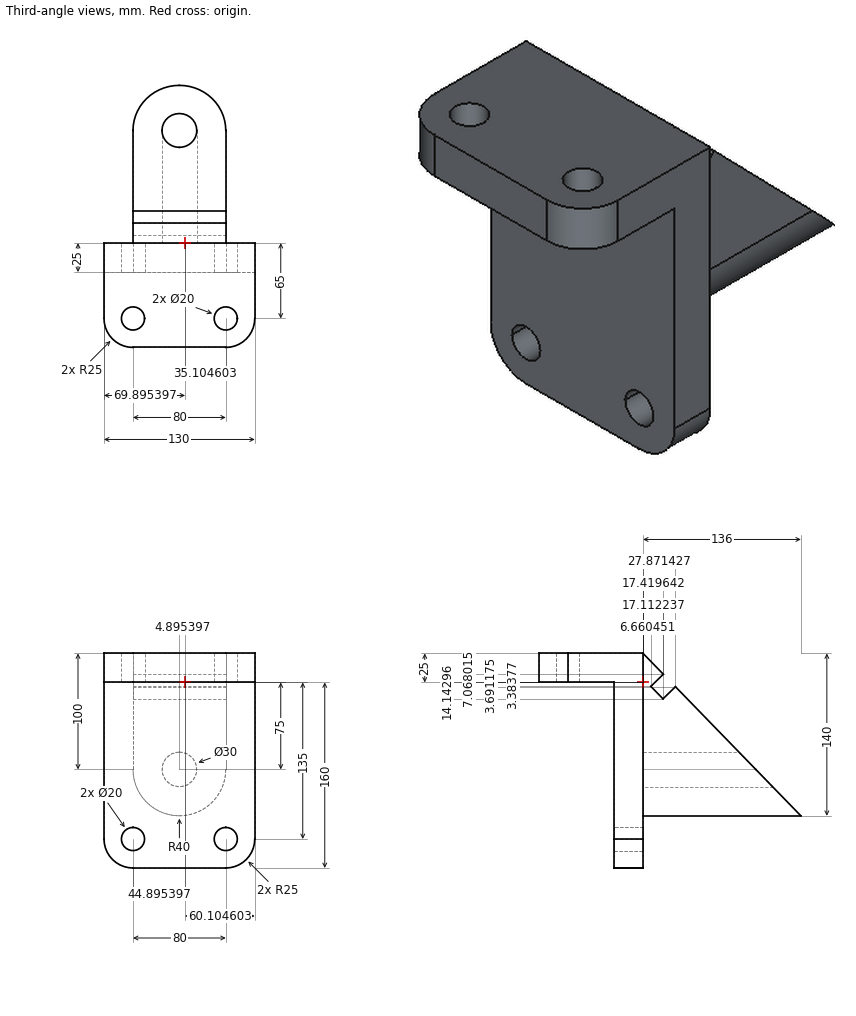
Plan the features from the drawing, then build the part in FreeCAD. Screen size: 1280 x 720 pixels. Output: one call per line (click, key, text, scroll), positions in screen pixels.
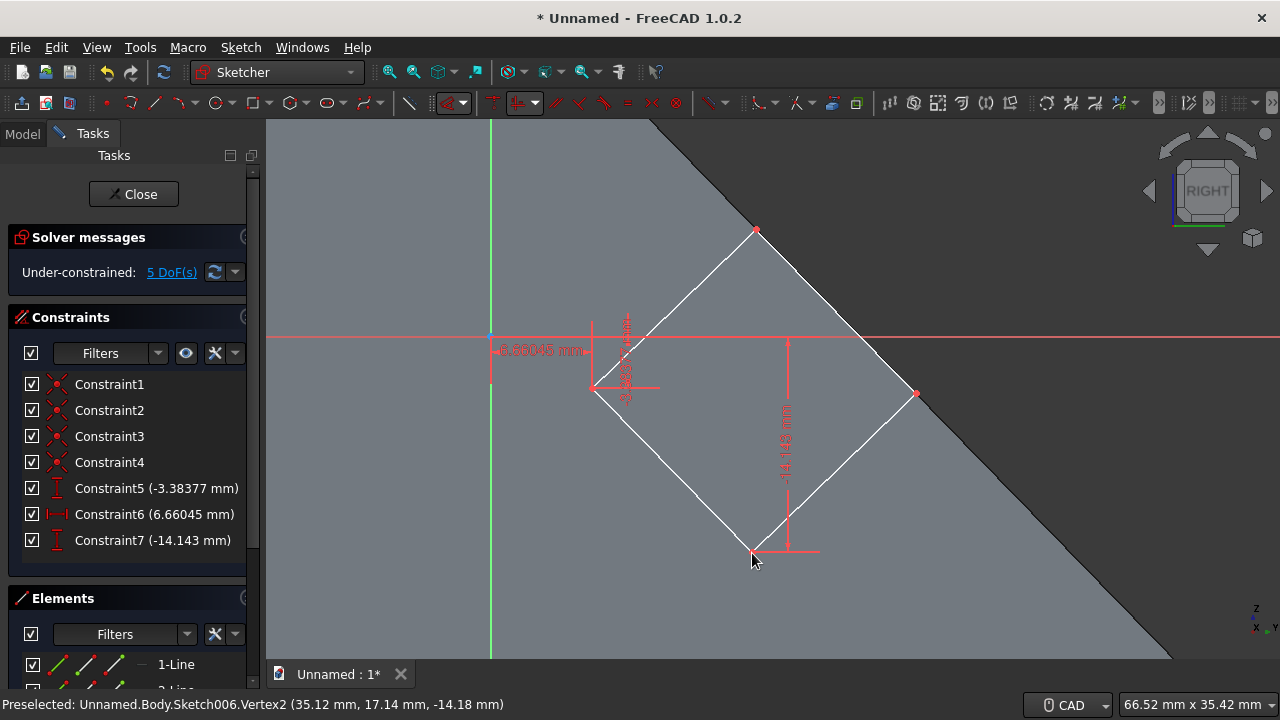
click(916, 394)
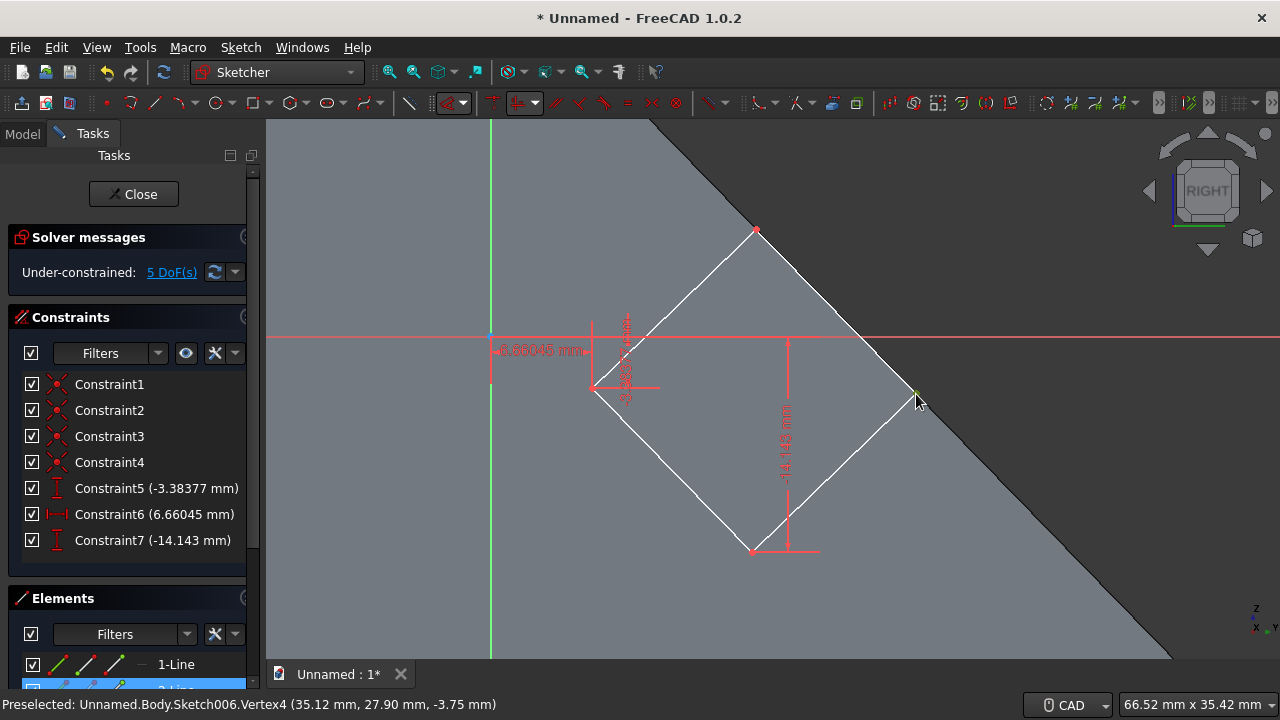
key(i)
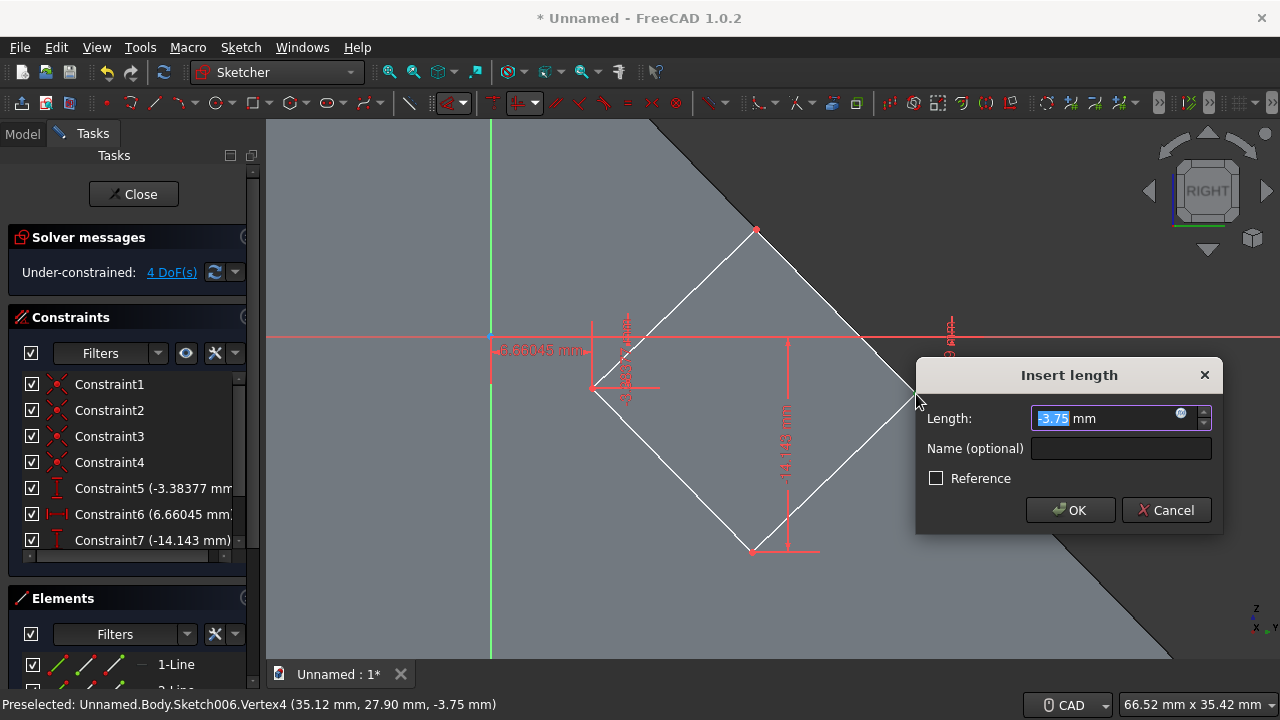
text(-3.691175)
key(Return)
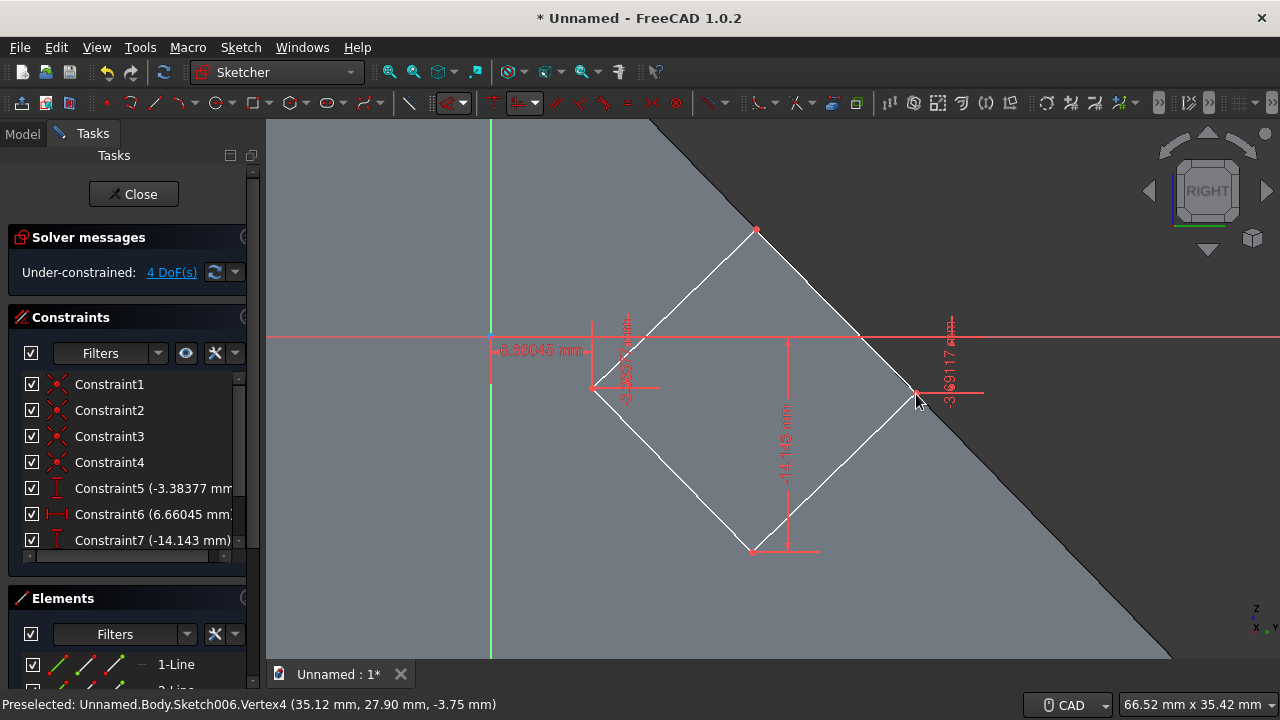
click(756, 230)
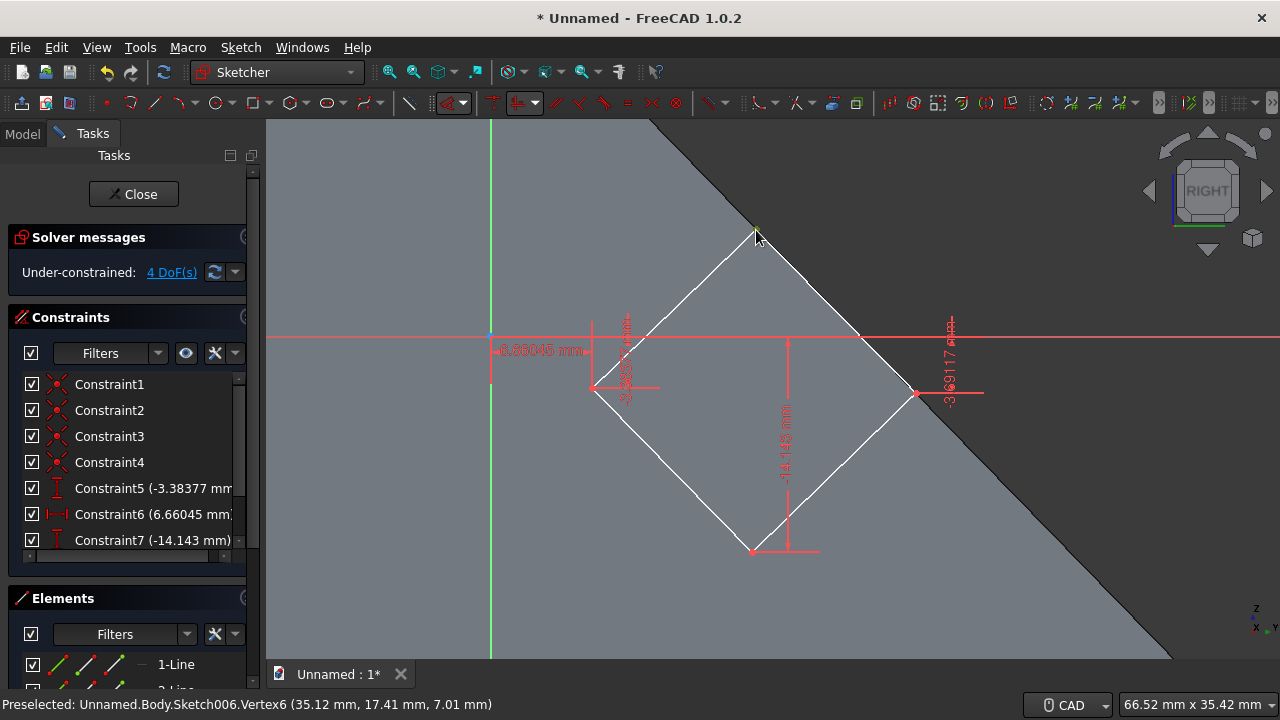
click(466, 104)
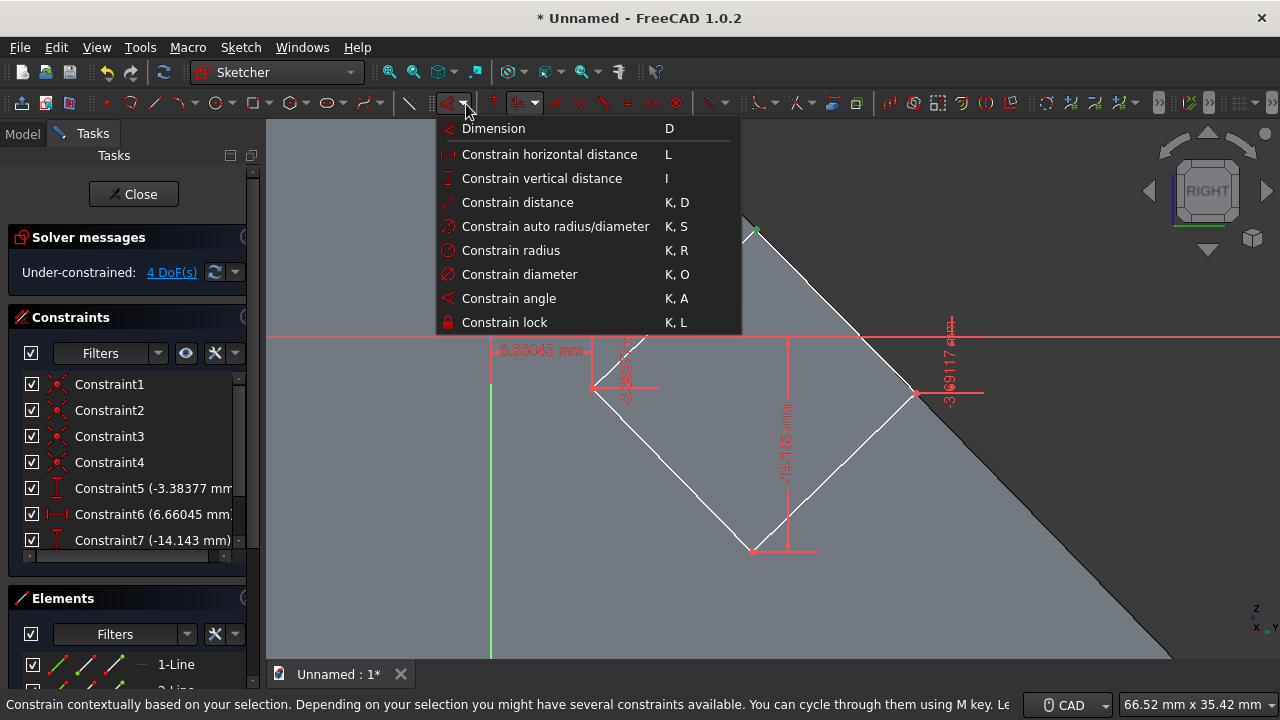
click(589, 178)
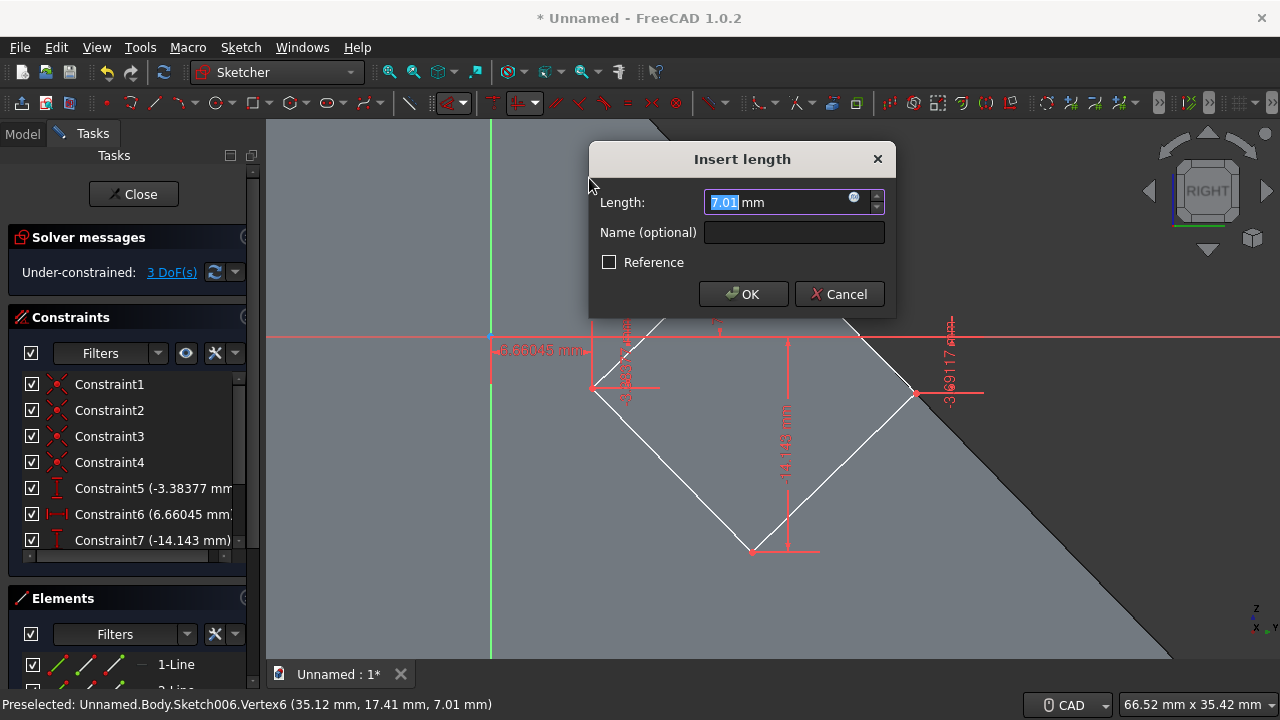
text(7.068015)
key(Return)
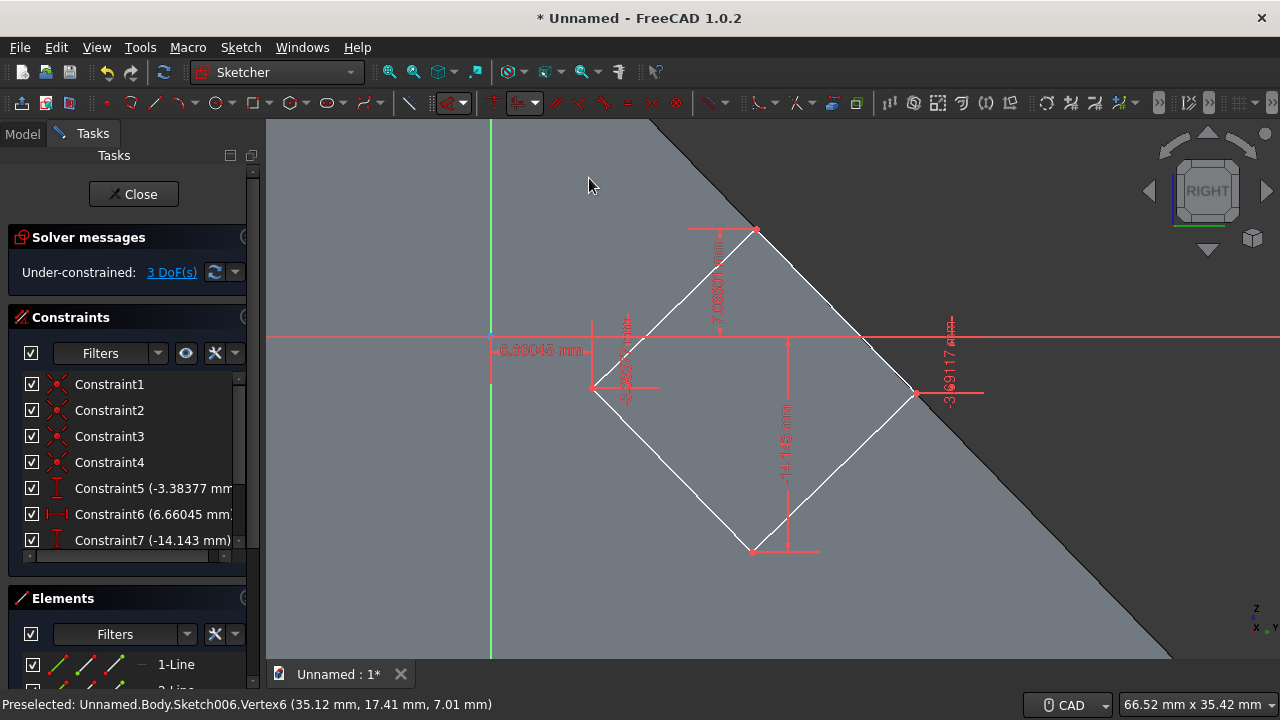
click(752, 552)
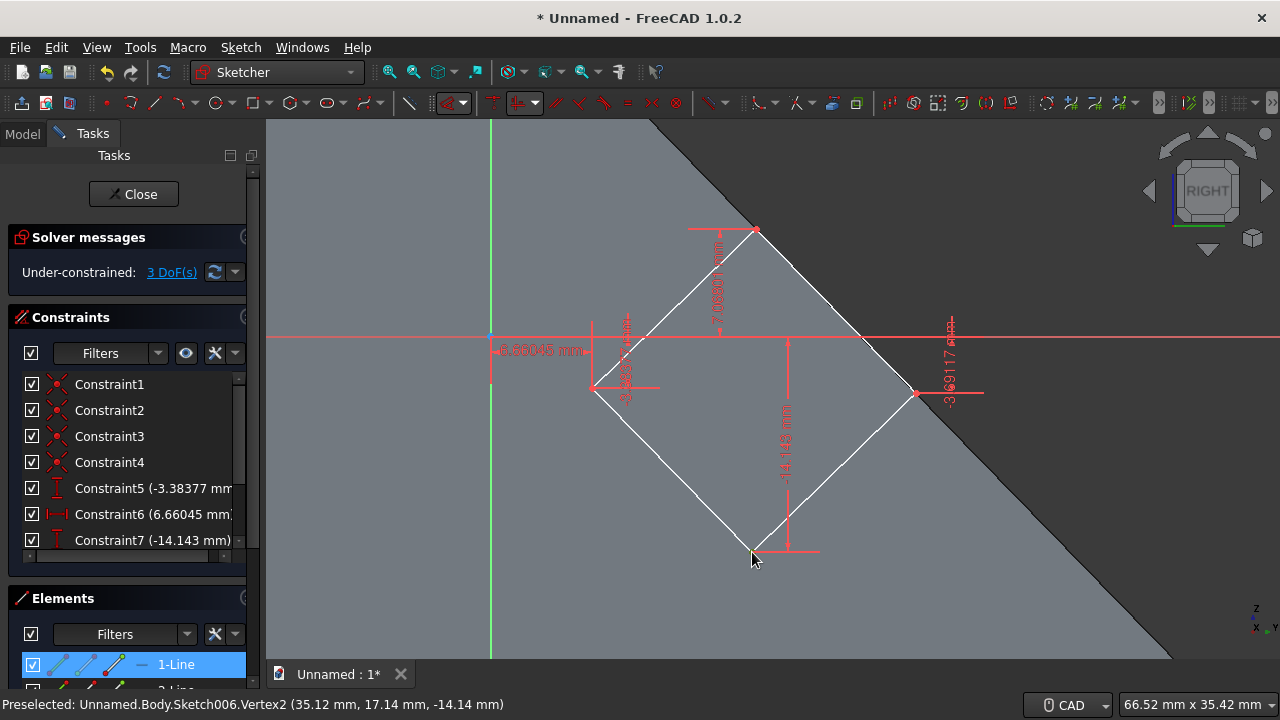
click(466, 104)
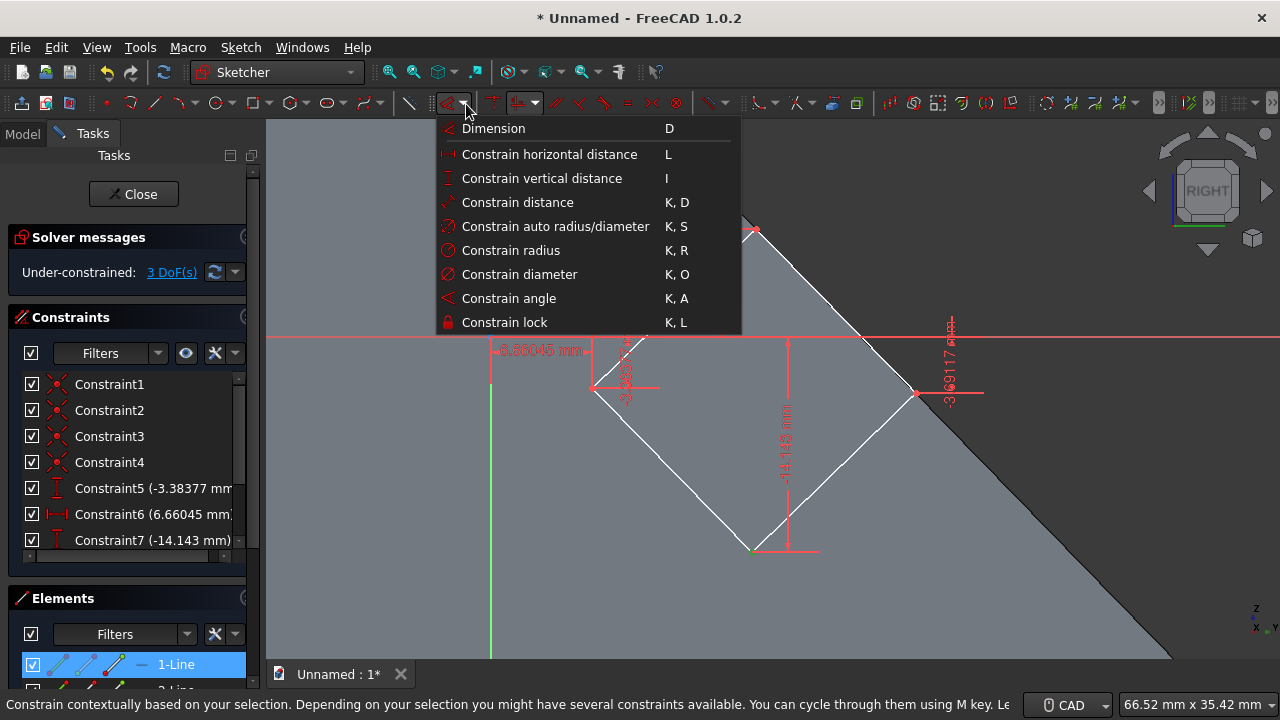
click(589, 154)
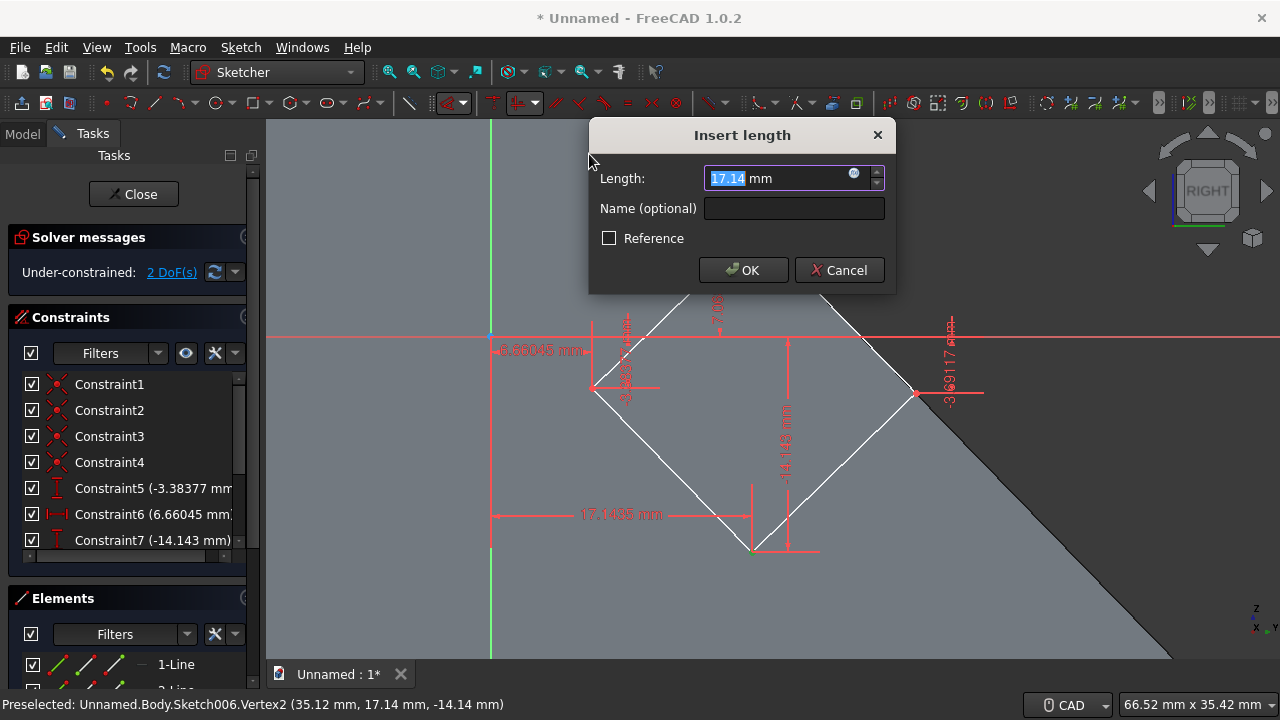
text(17.112237)
key(Return)